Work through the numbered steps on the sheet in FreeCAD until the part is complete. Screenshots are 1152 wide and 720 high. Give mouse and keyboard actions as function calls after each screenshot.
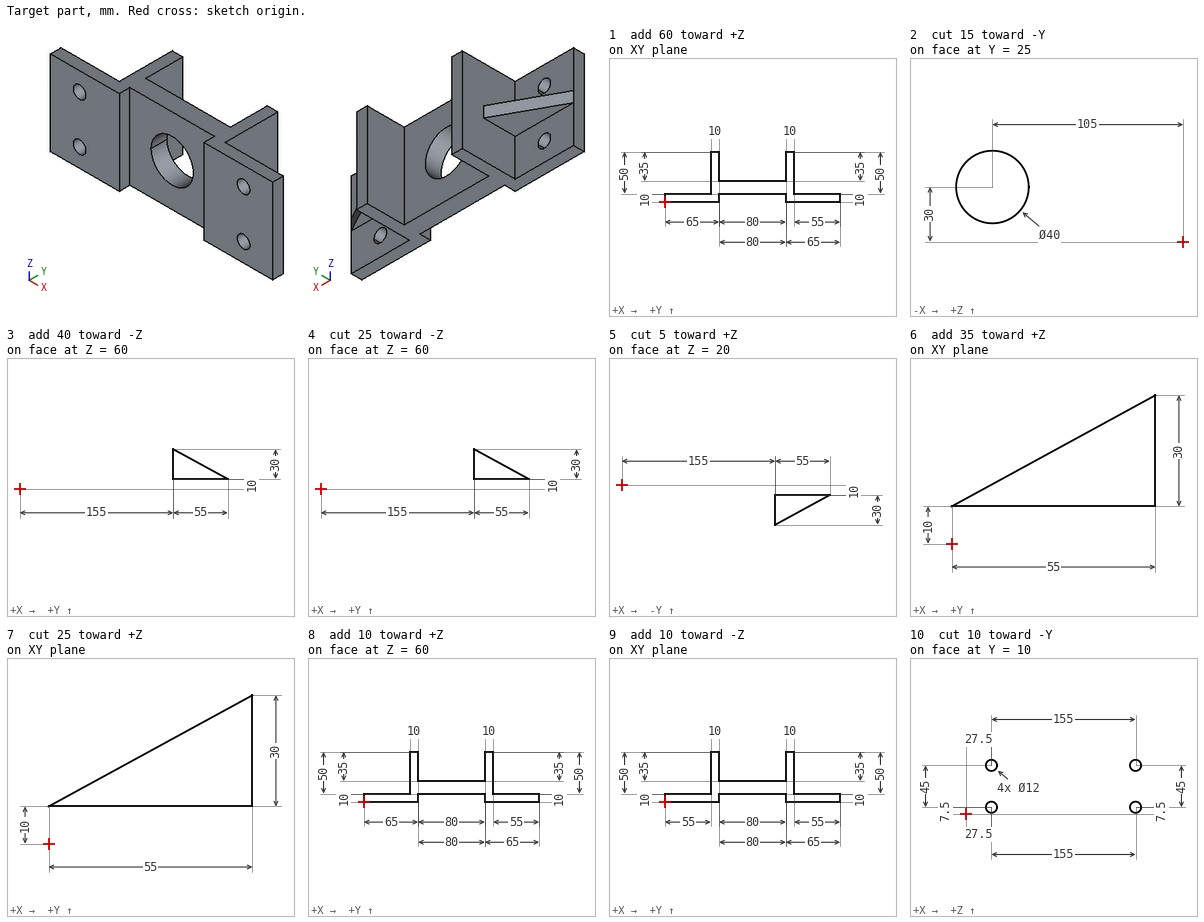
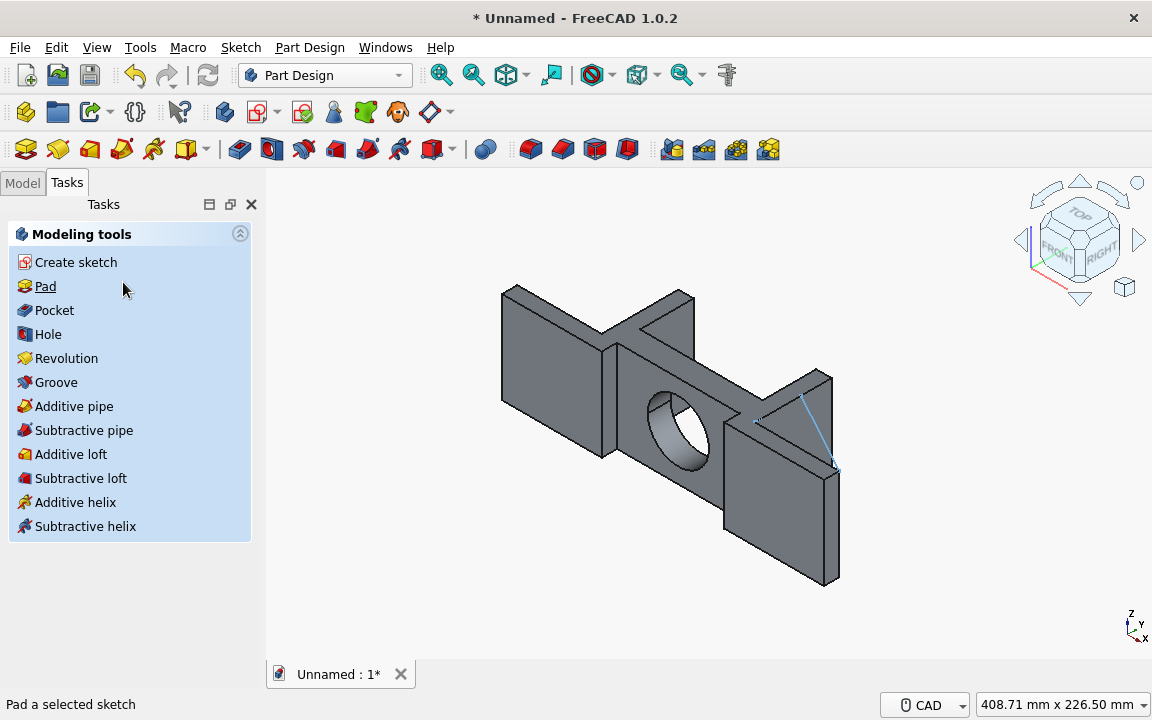
click(26, 150)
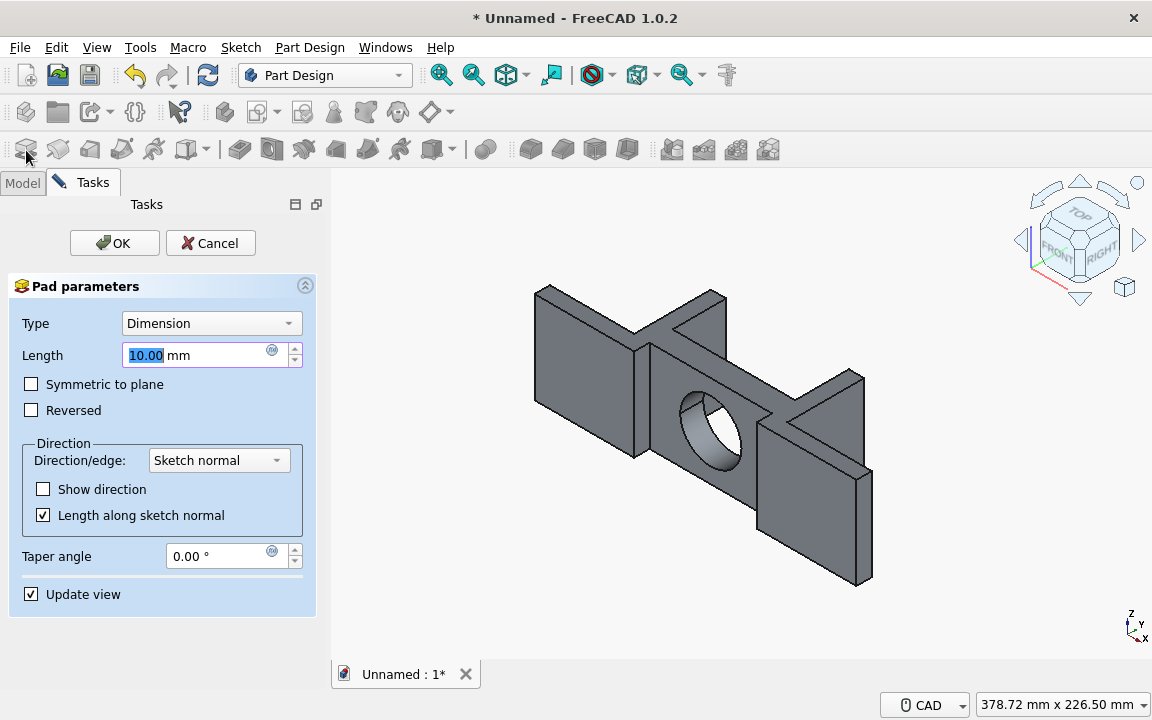
text(40)
key(Tab)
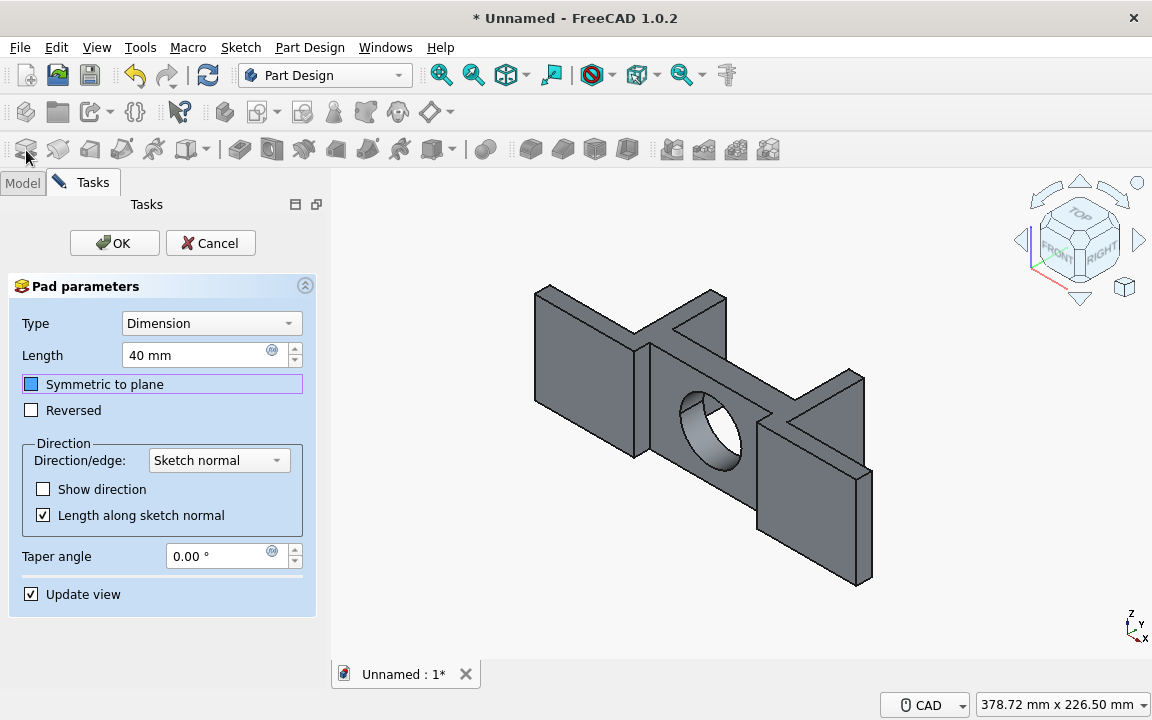
click(30, 410)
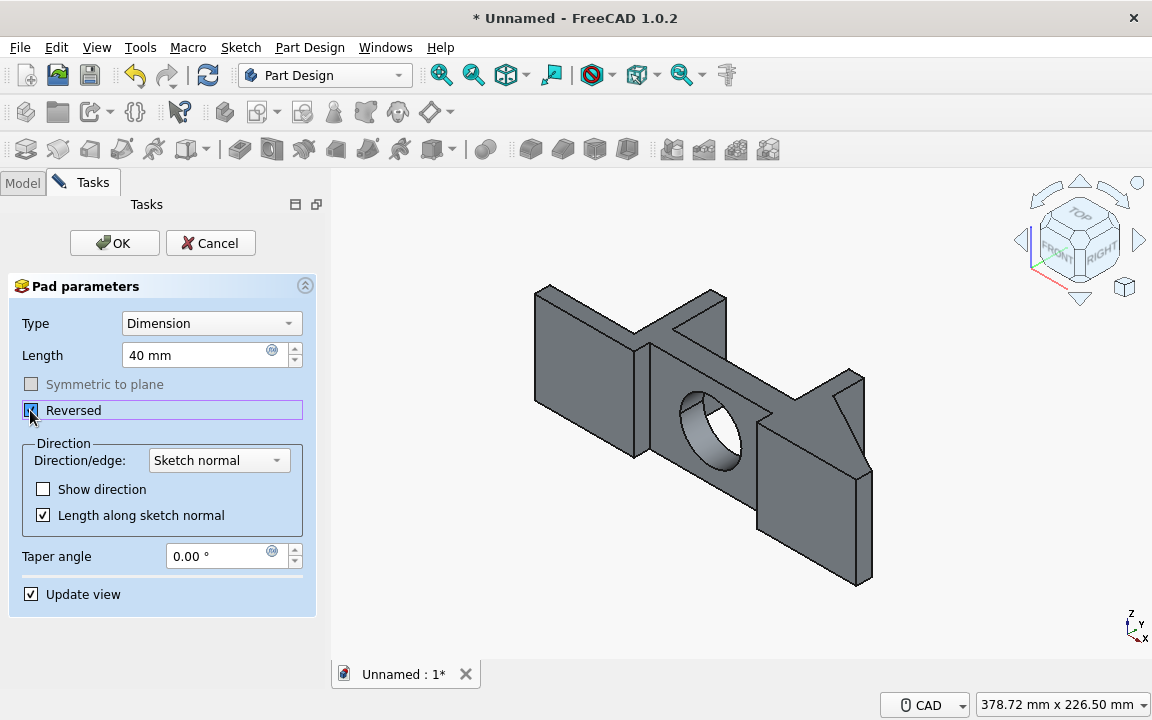
click(115, 243)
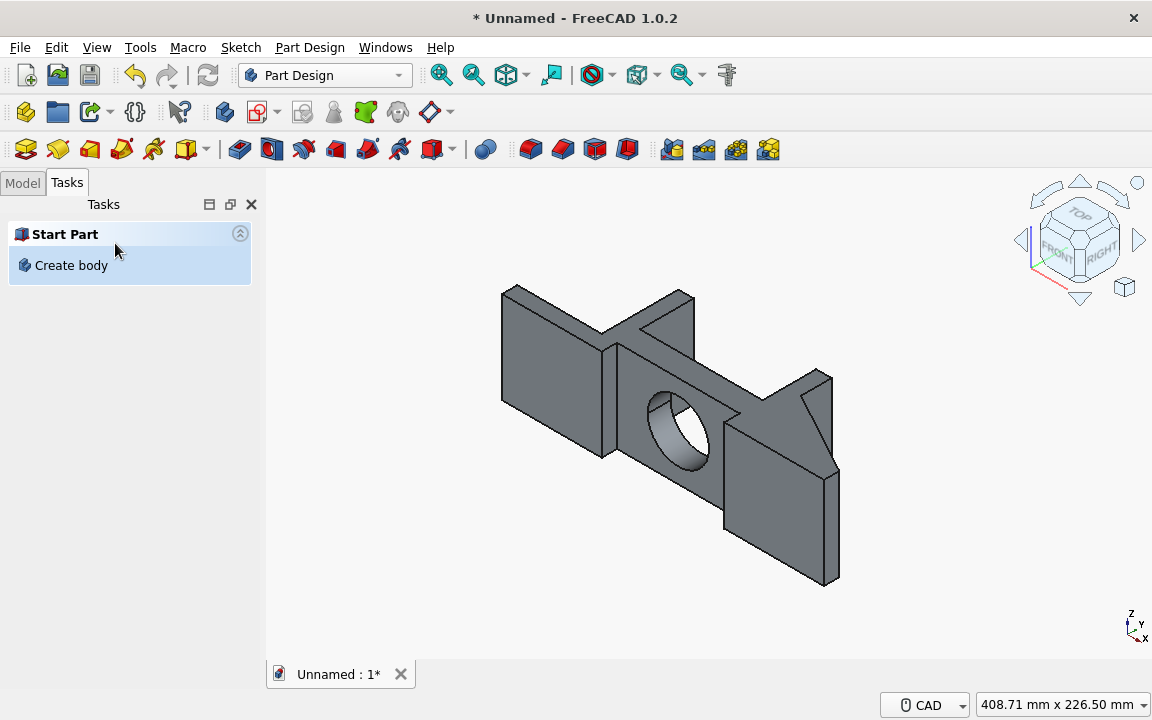
click(775, 428)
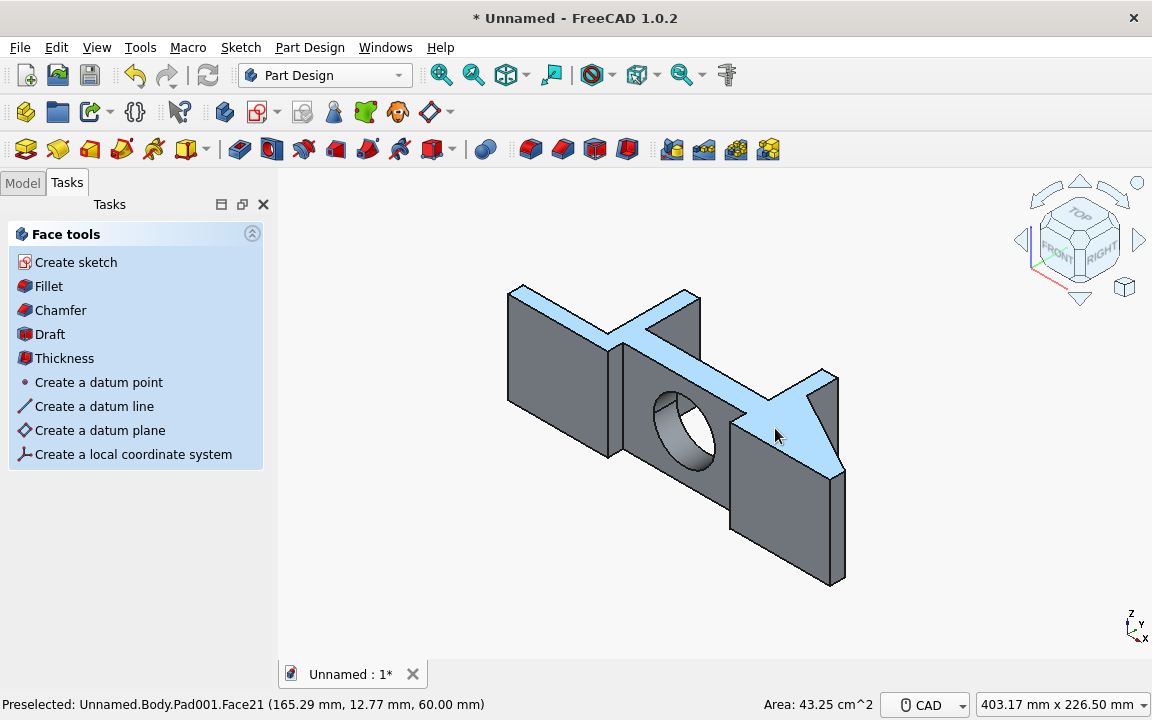
click(258, 112)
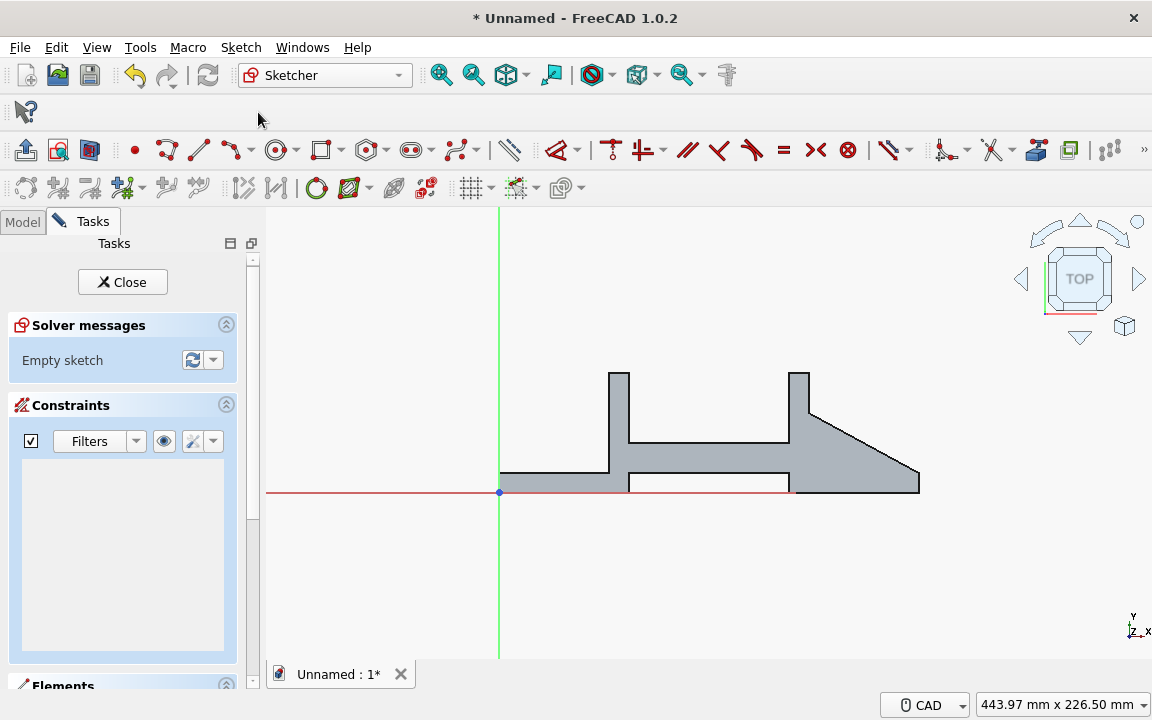
scroll(937, 446, up, 7)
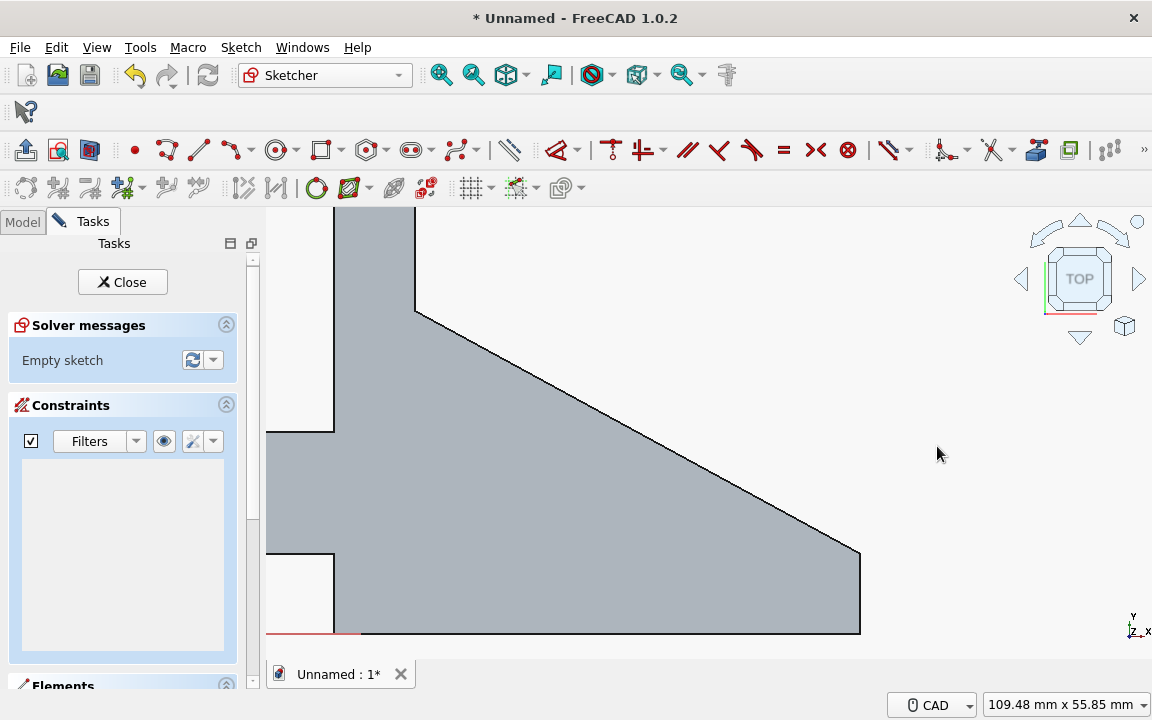
key(g)
key(m)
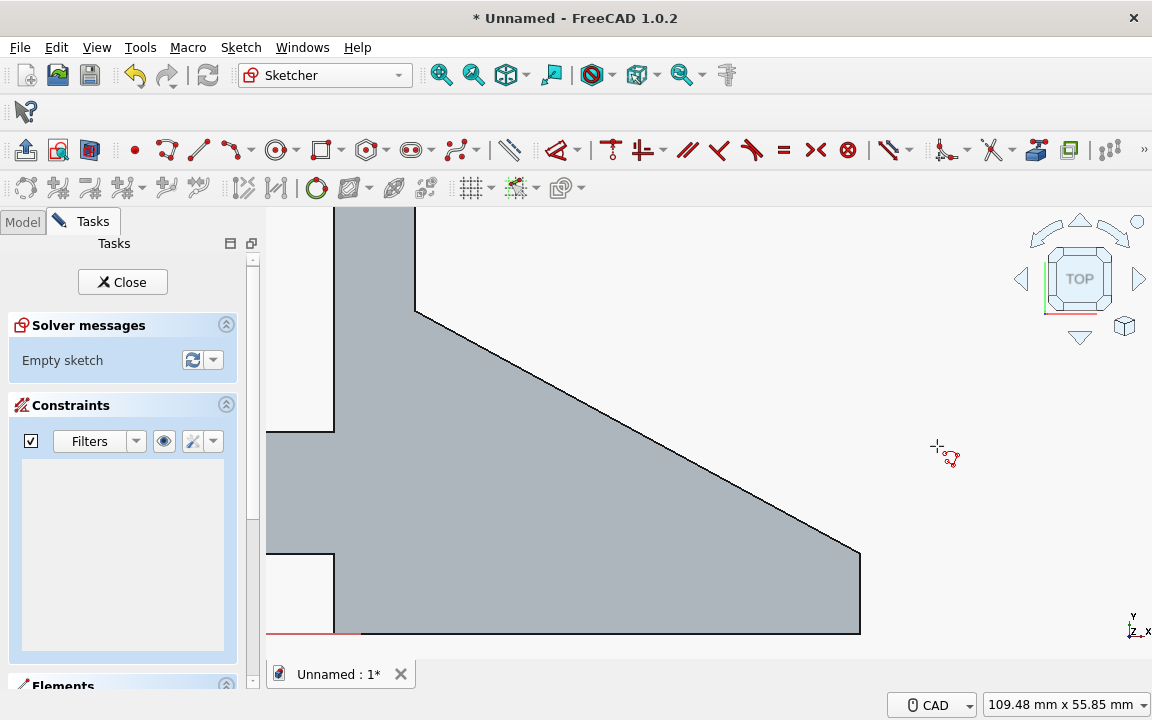
click(415, 554)
click(860, 554)
click(415, 311)
click(415, 555)
key(Escape)
key(Escape)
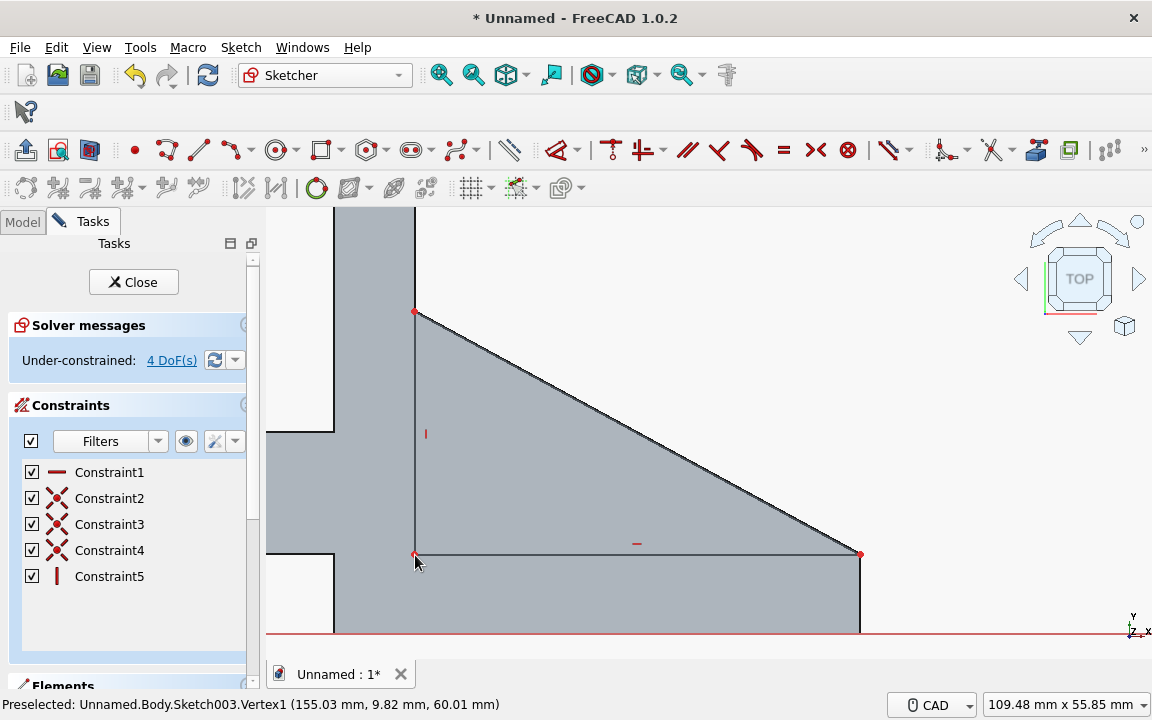
key(d)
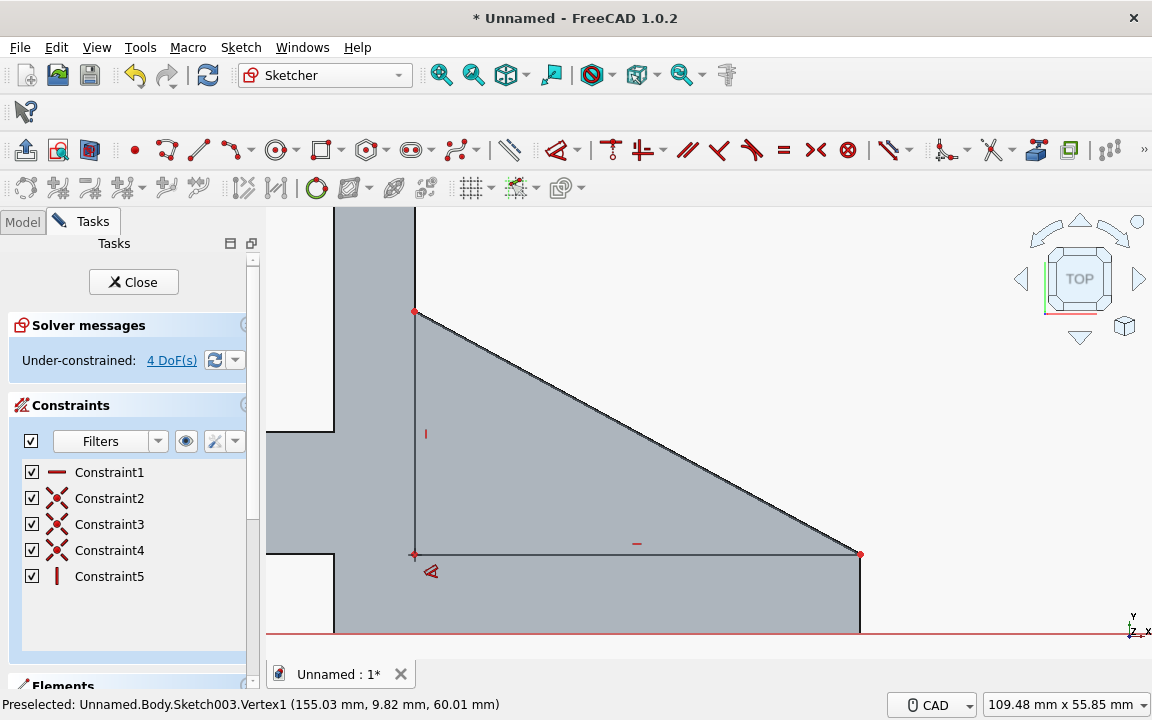
click(548, 555)
click(637, 589)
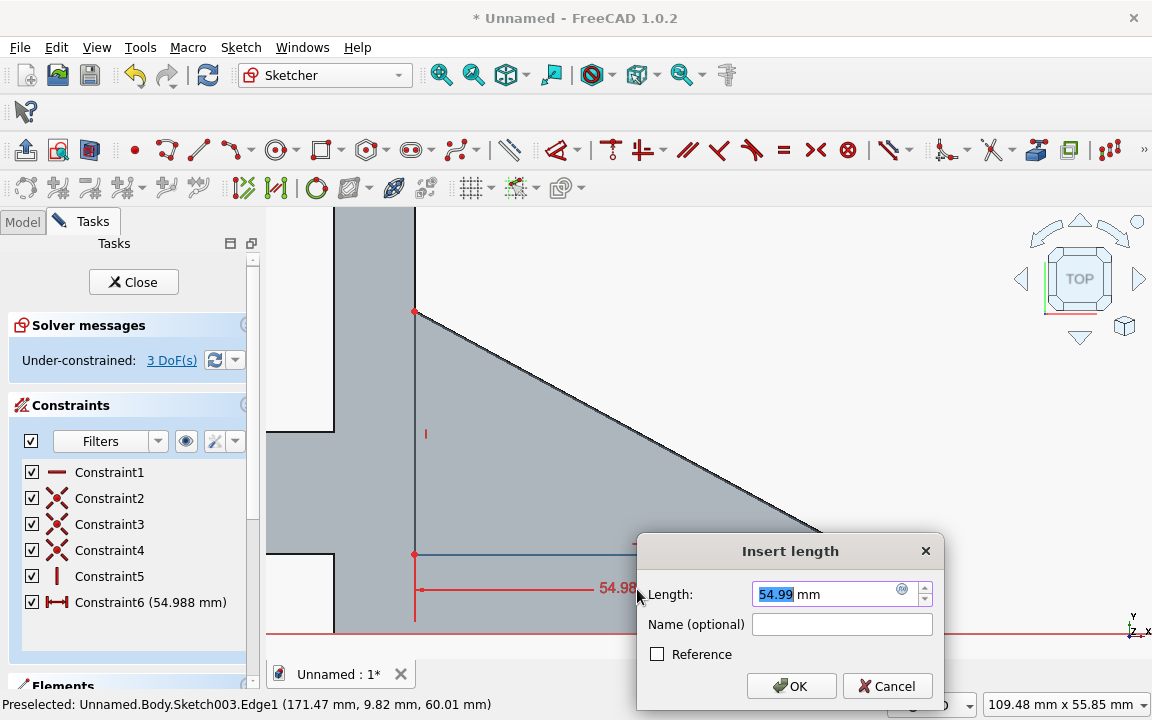
text(55)
key(Return)